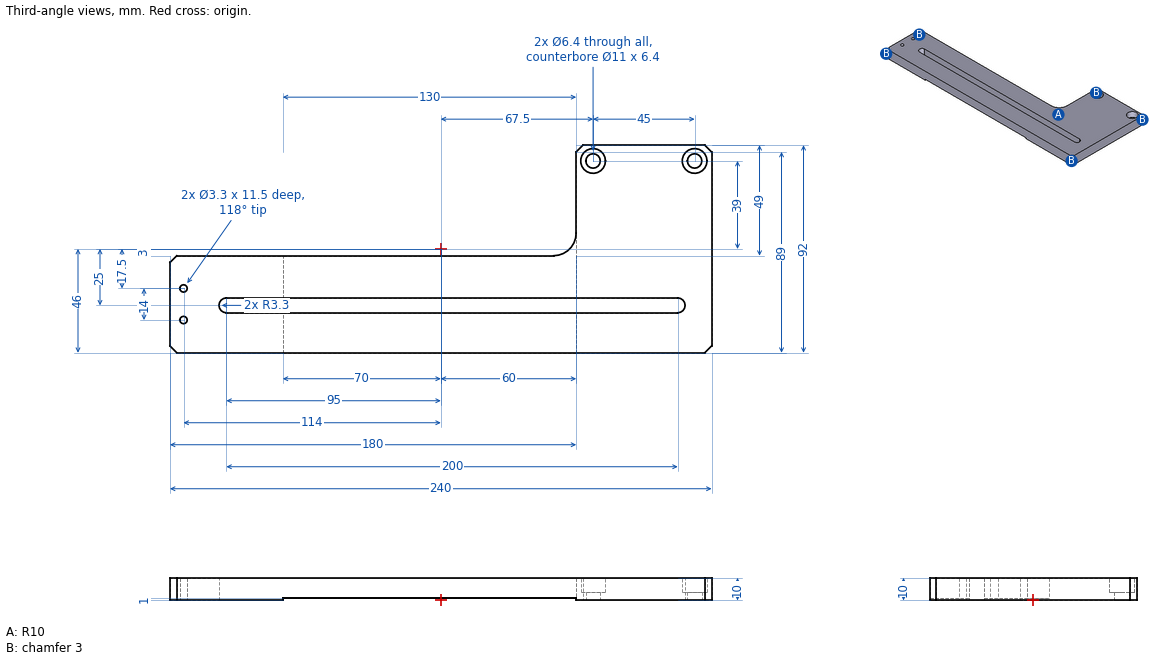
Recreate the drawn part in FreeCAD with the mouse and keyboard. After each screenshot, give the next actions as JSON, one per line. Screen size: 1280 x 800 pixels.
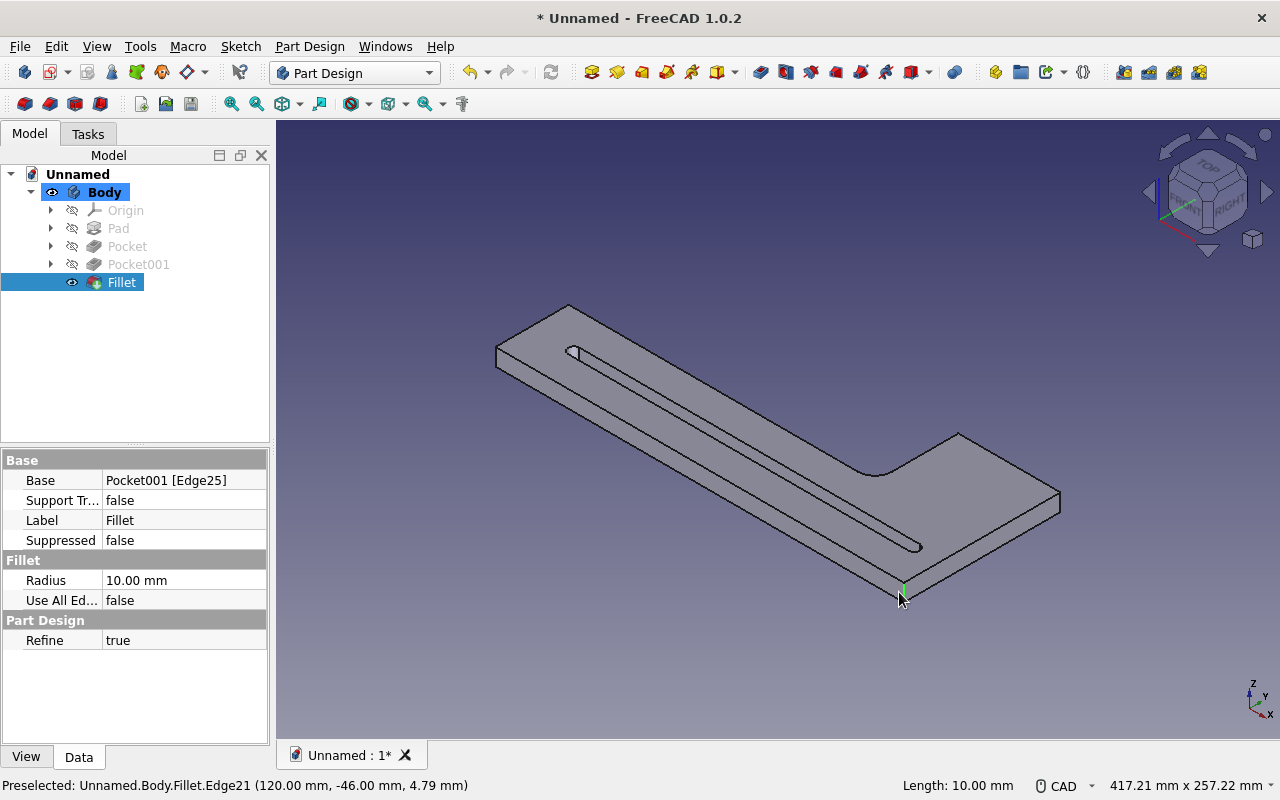
{"action": "key", "text": "1"}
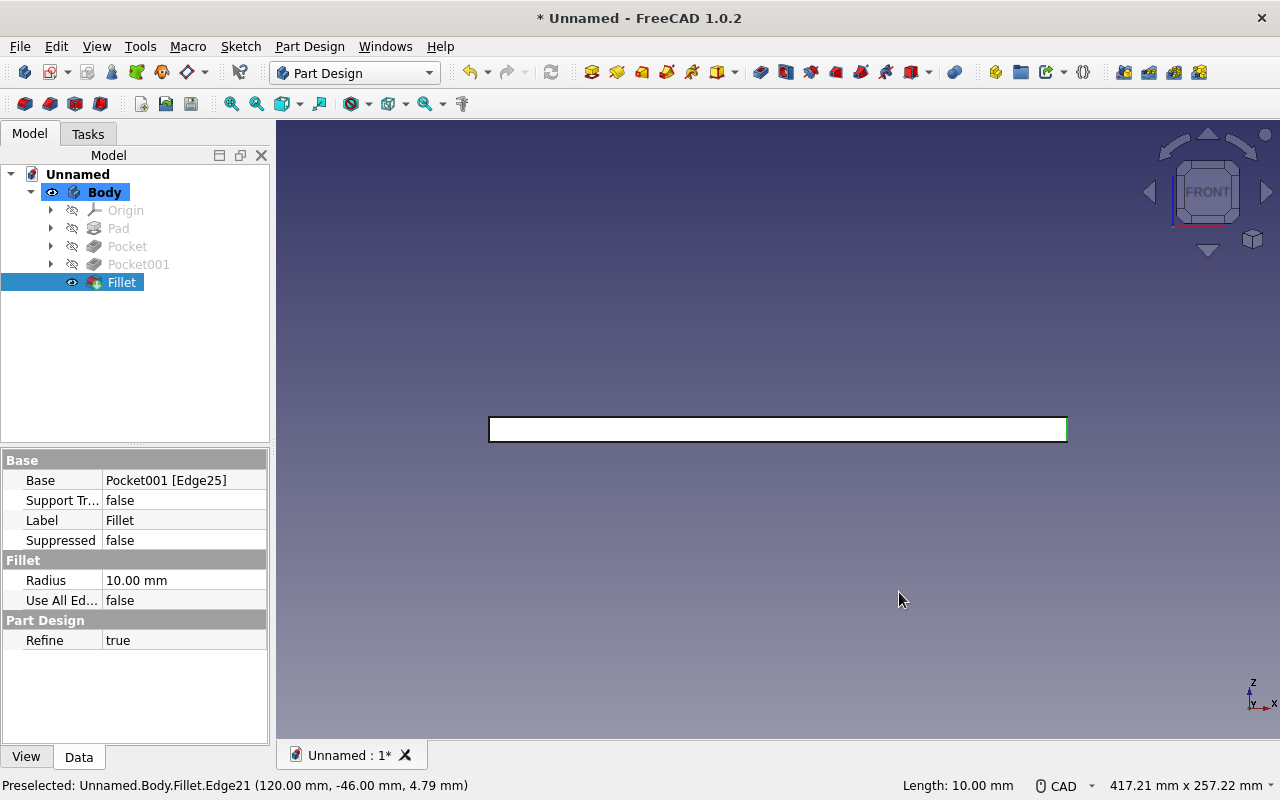
{"action": "left_click", "coordinate": [489, 429], "text": "ctrl"}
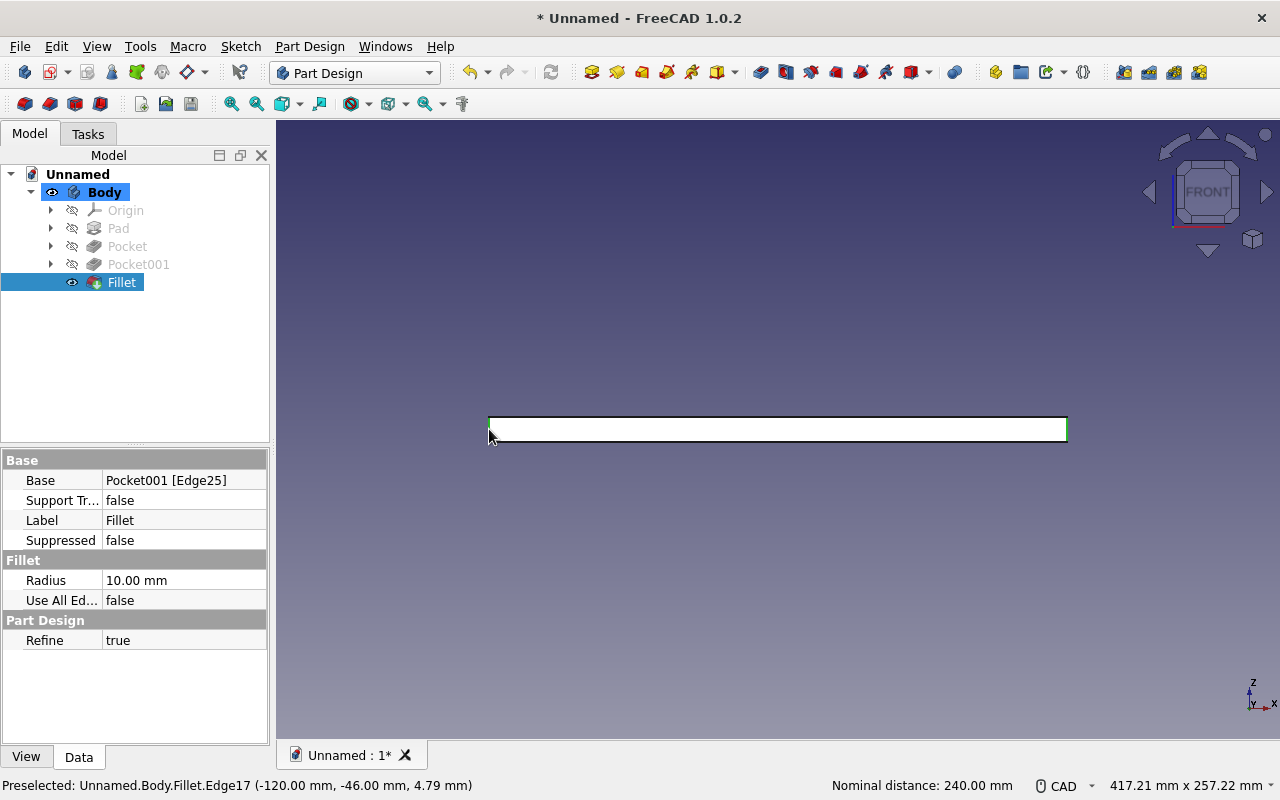
{"action": "key", "text": "3"}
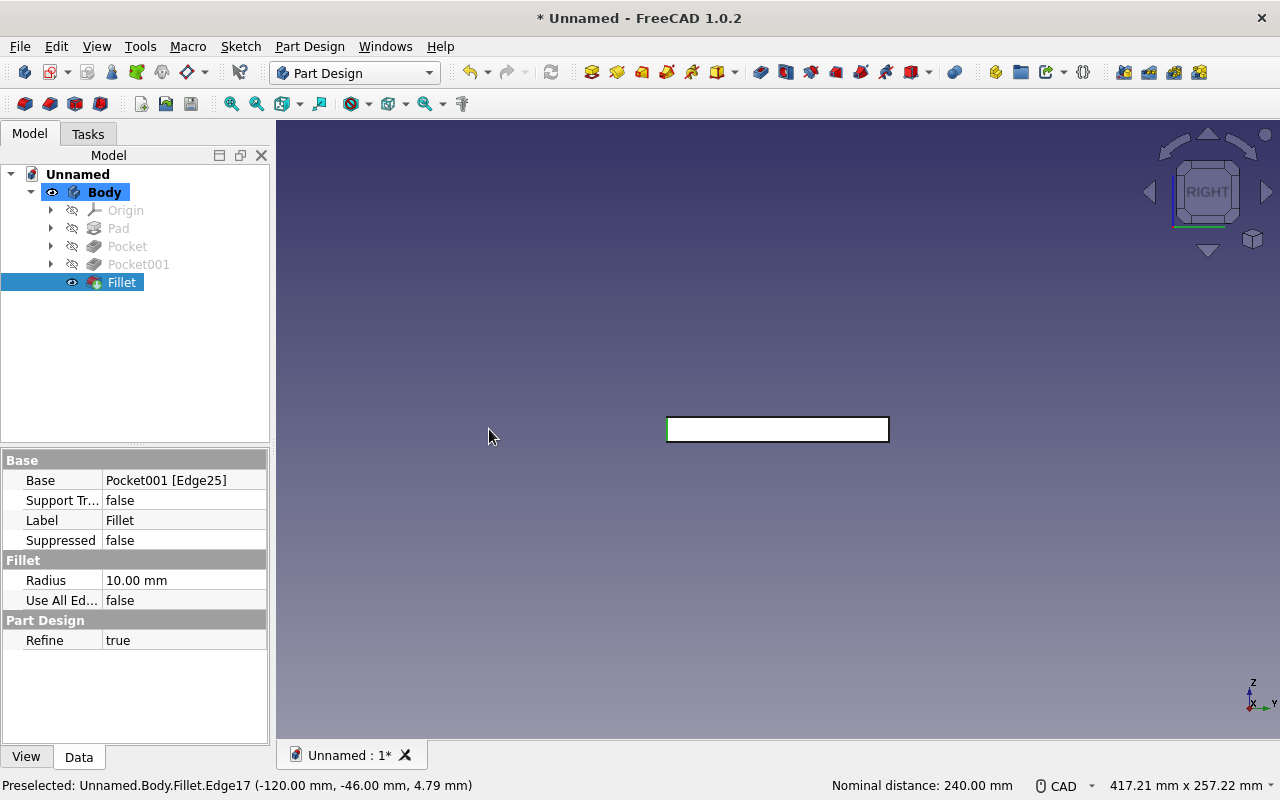
{"action": "key", "text": "v f"}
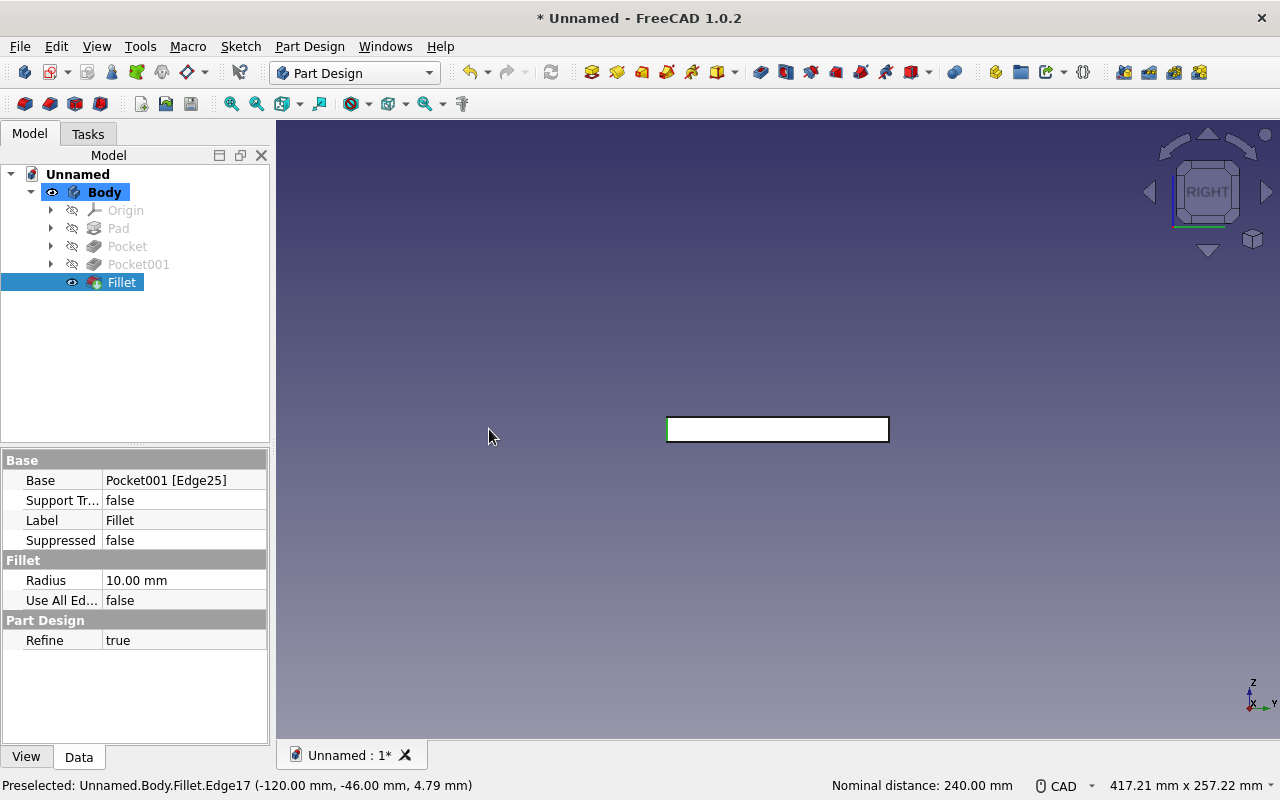
{"action": "left_click", "coordinate": [889, 428], "text": "ctrl"}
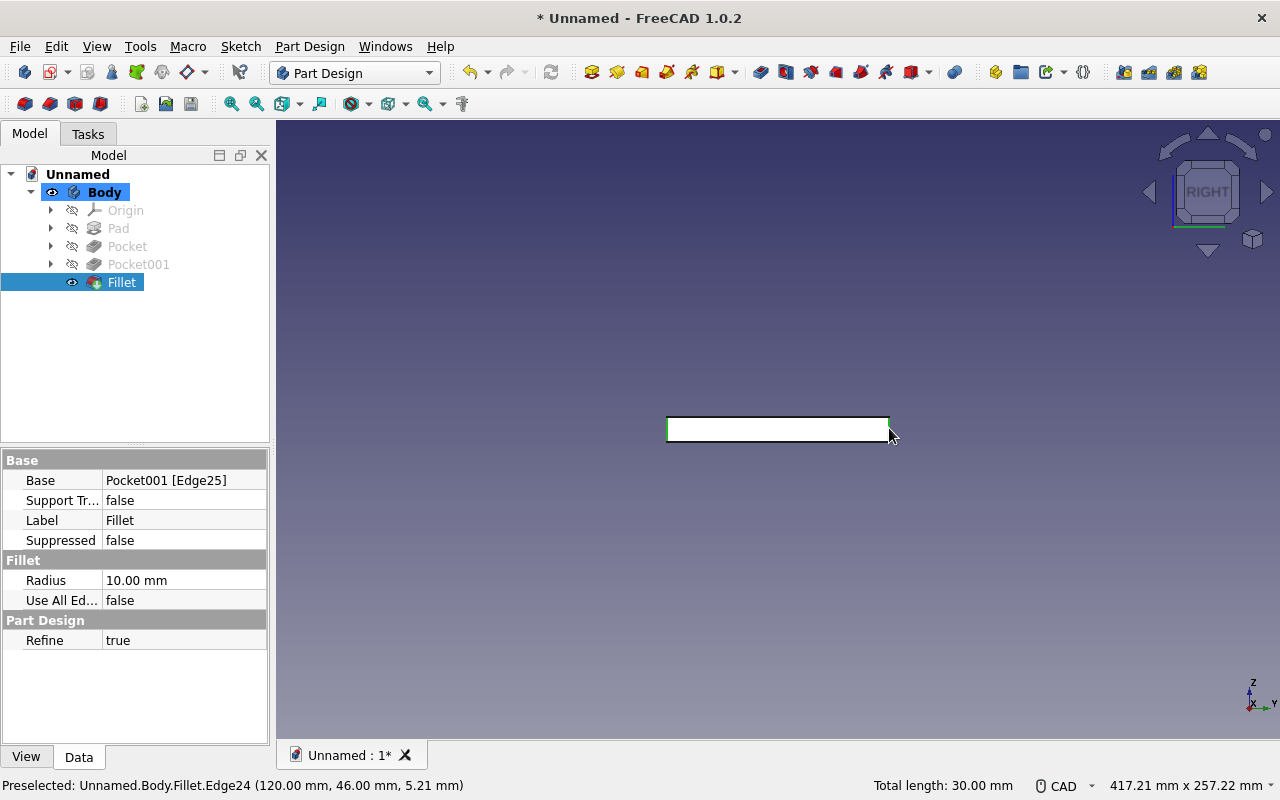
{"action": "key", "text": "5"}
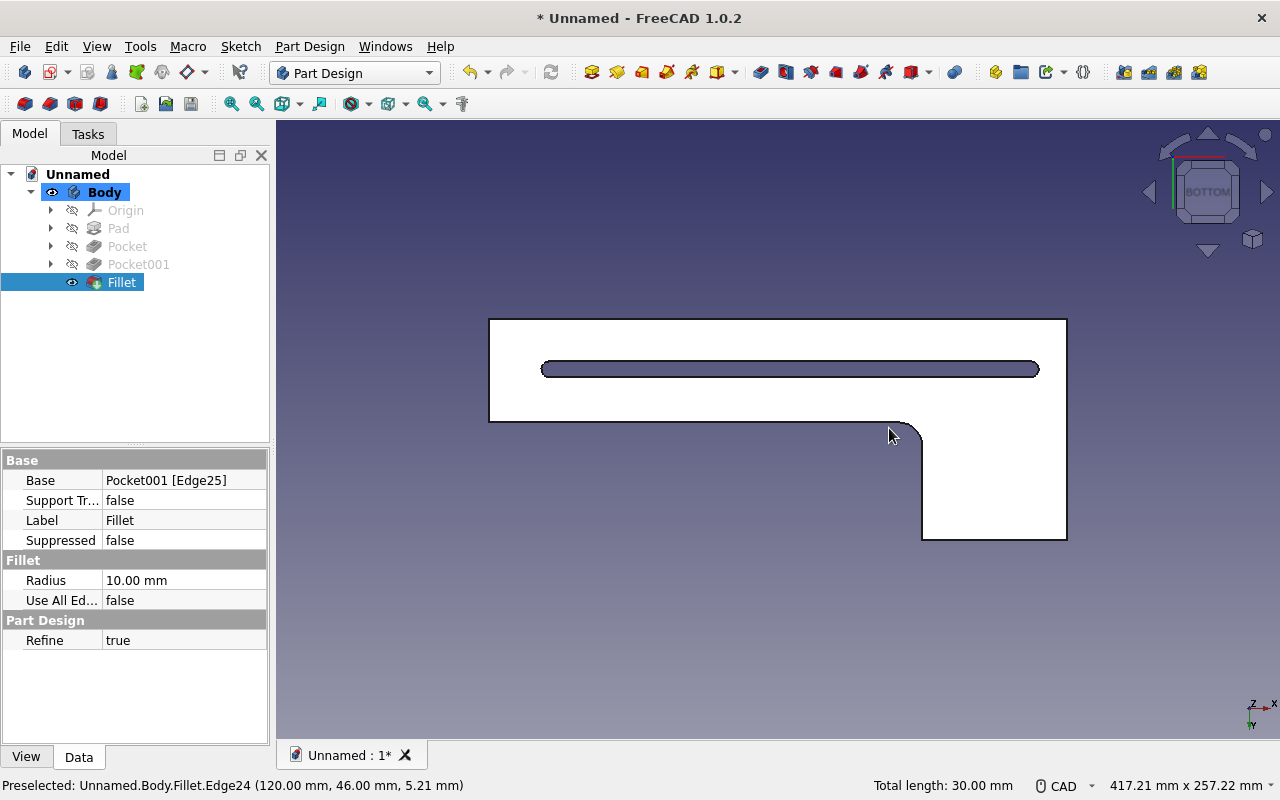
{"action": "key", "text": "4"}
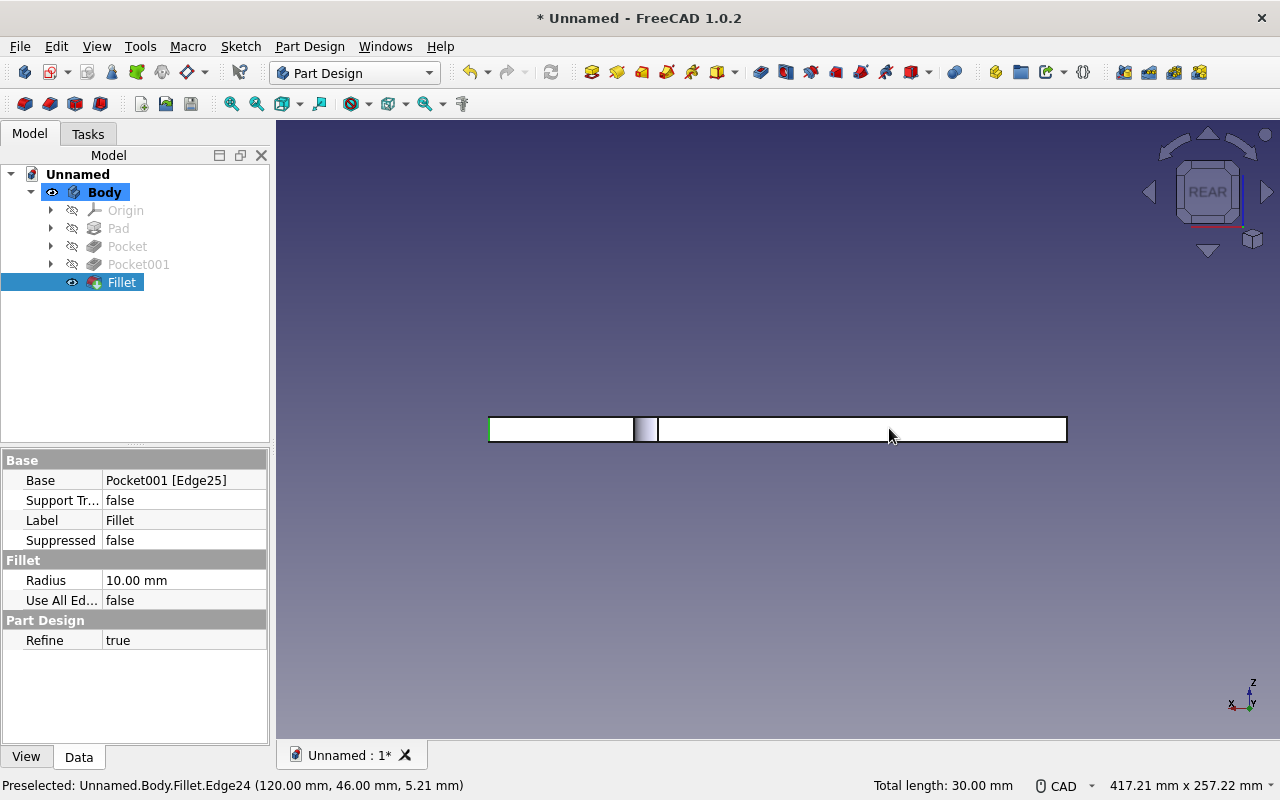
{"action": "left_click", "coordinate": [1067, 429], "text": "ctrl"}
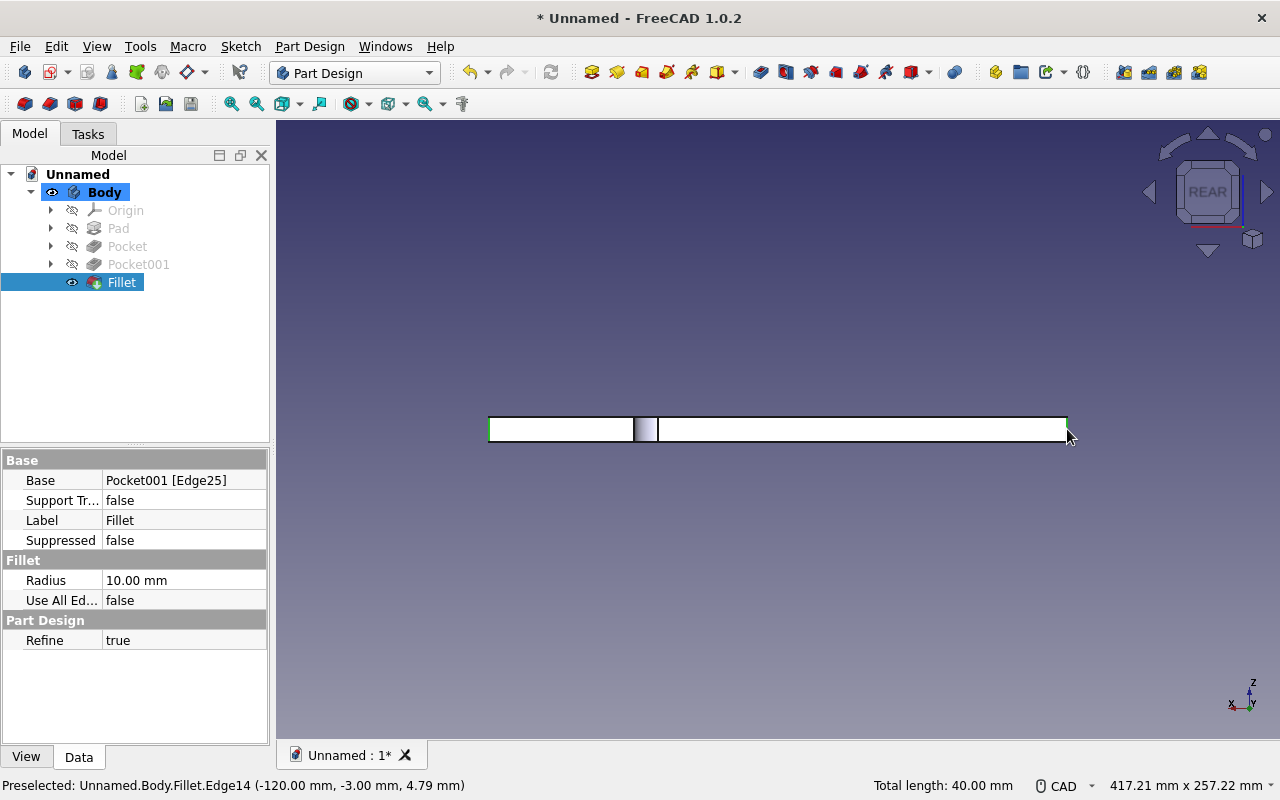
{"action": "left_click", "coordinate": [634, 429], "text": "ctrl"}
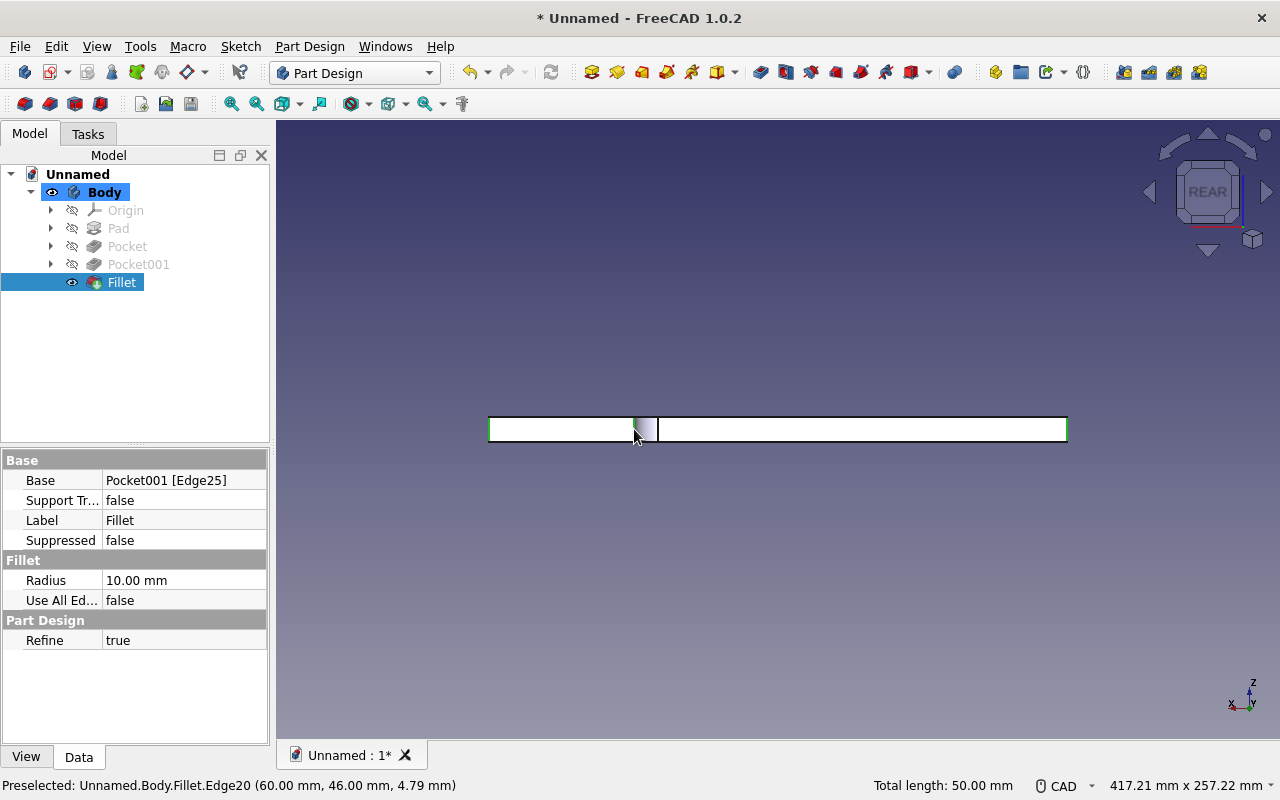
{"action": "left_click", "coordinate": [50, 104]}